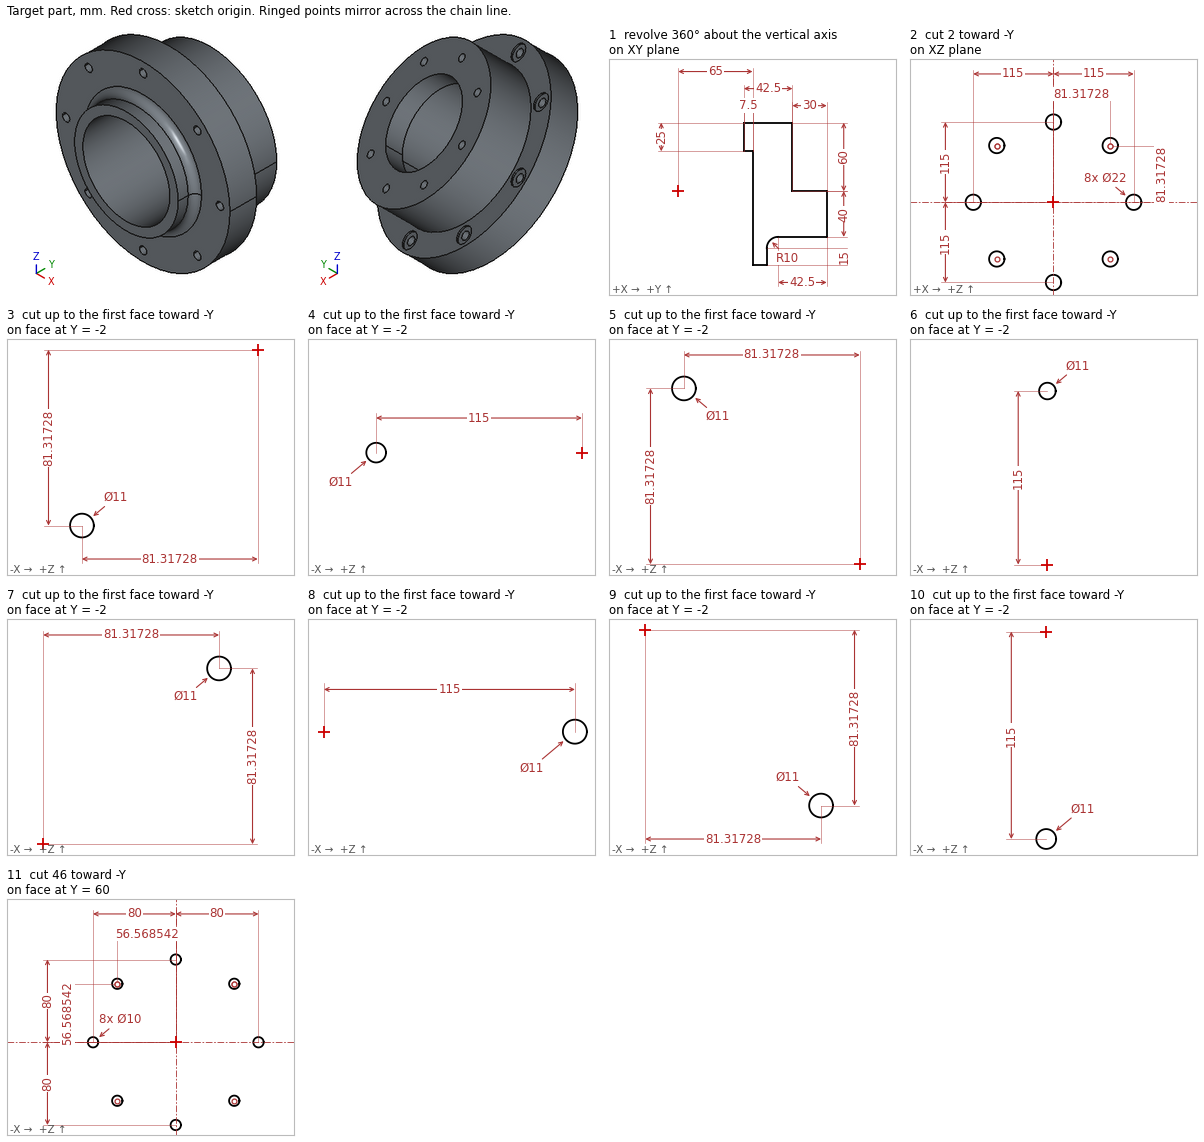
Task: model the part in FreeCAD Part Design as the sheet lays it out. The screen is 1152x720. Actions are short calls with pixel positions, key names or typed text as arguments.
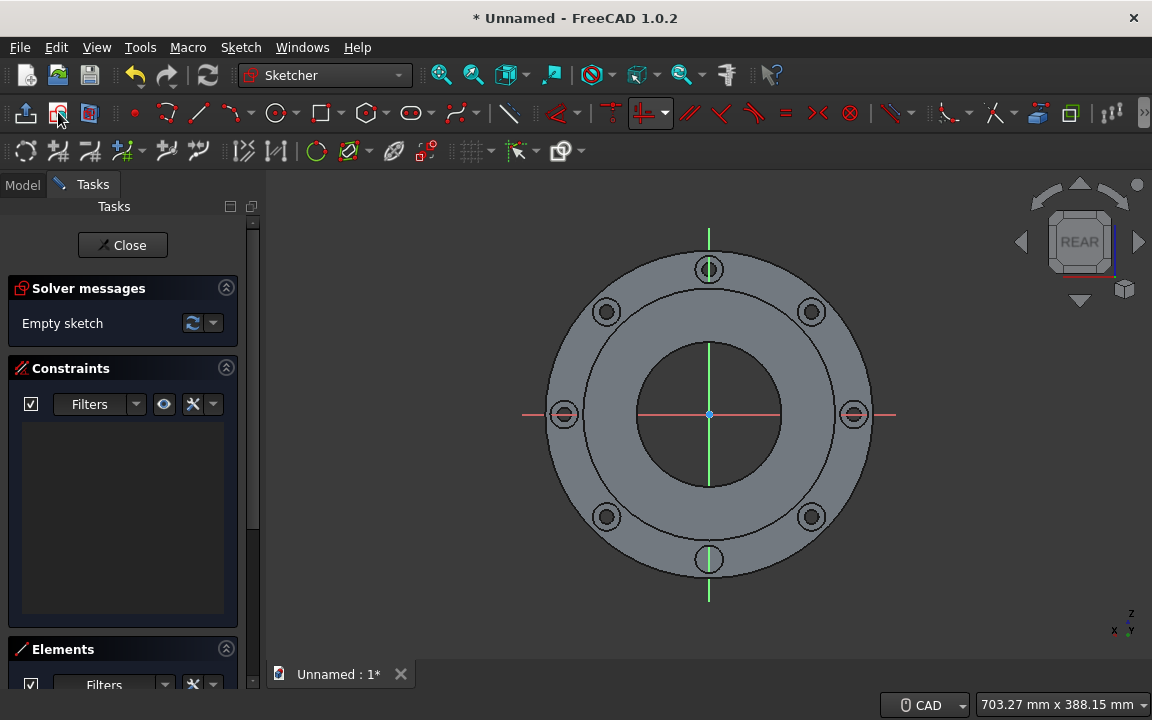
click(90, 114)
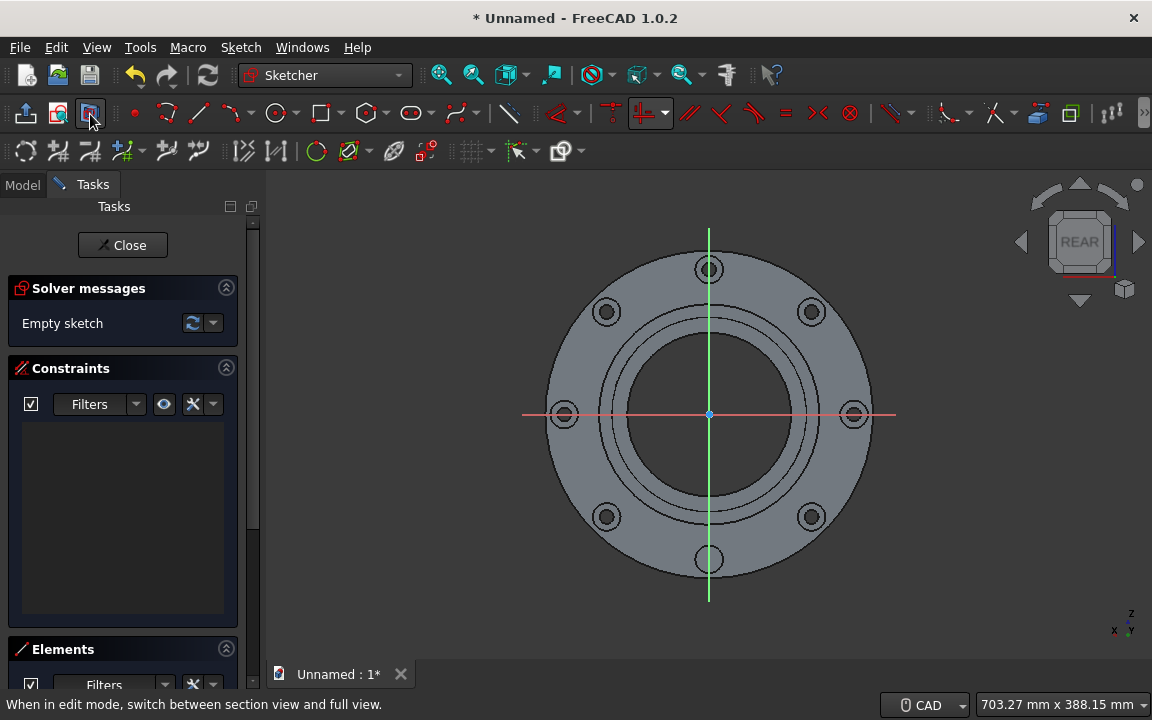
scroll(713, 567, up, 15)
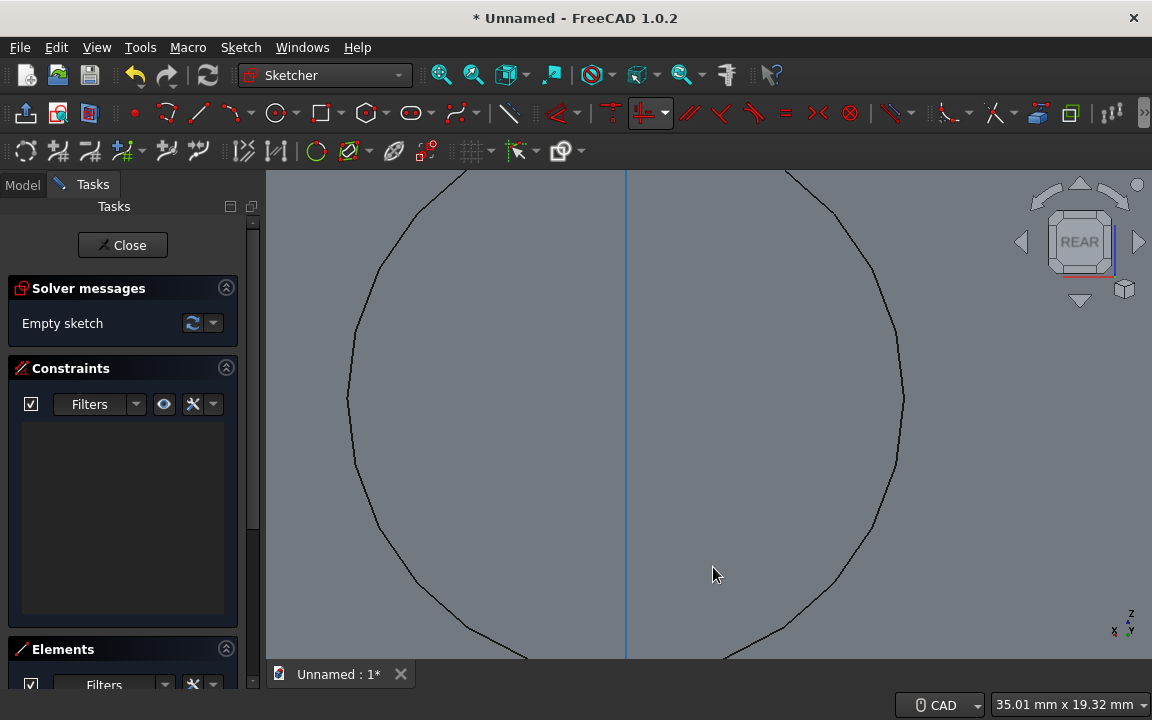
click(276, 114)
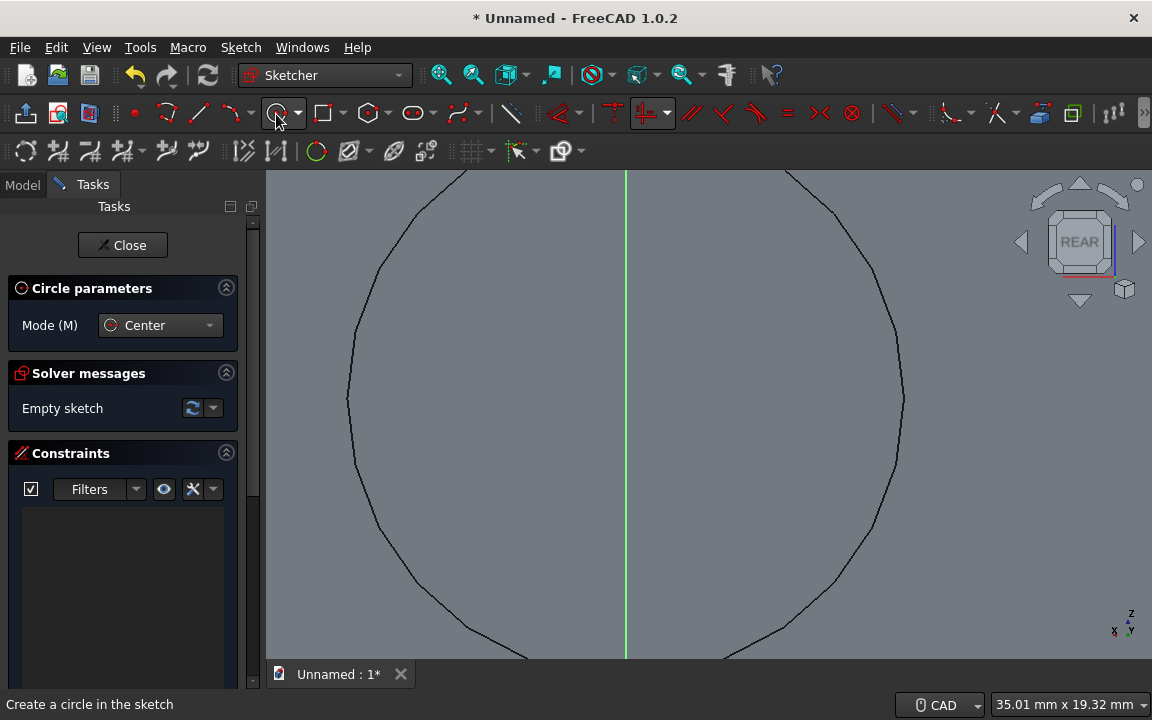
click(626, 398)
move(724, 300)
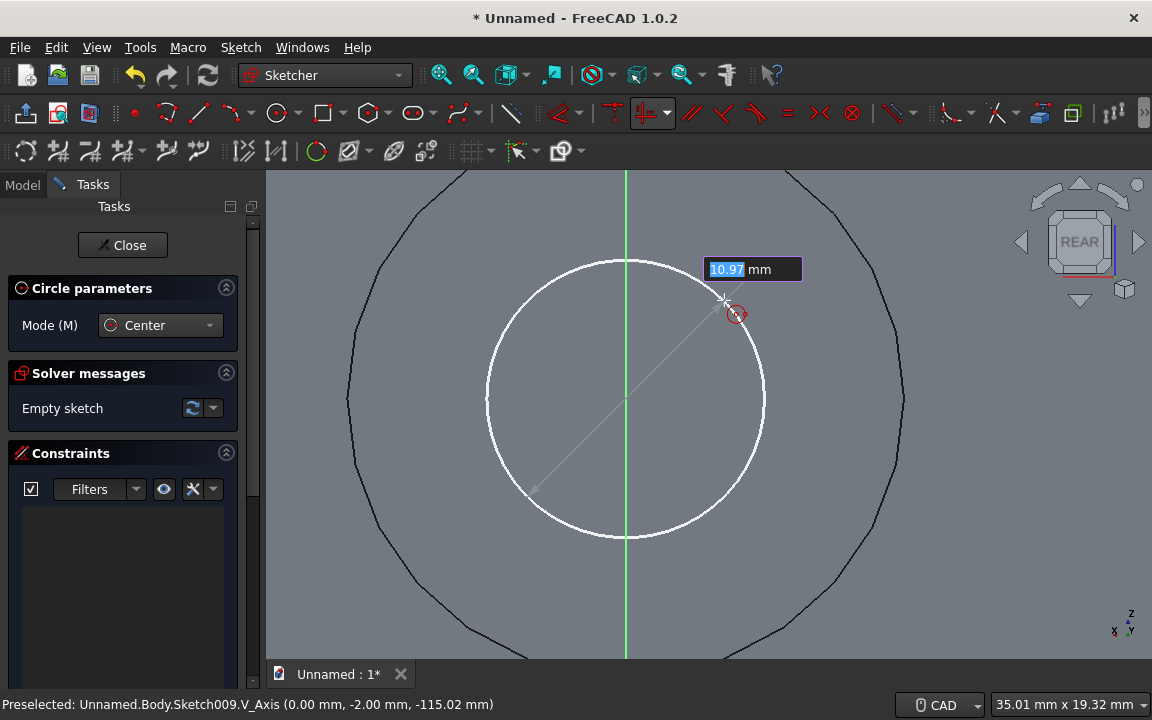
text(11)
key(Return)
key(Escape)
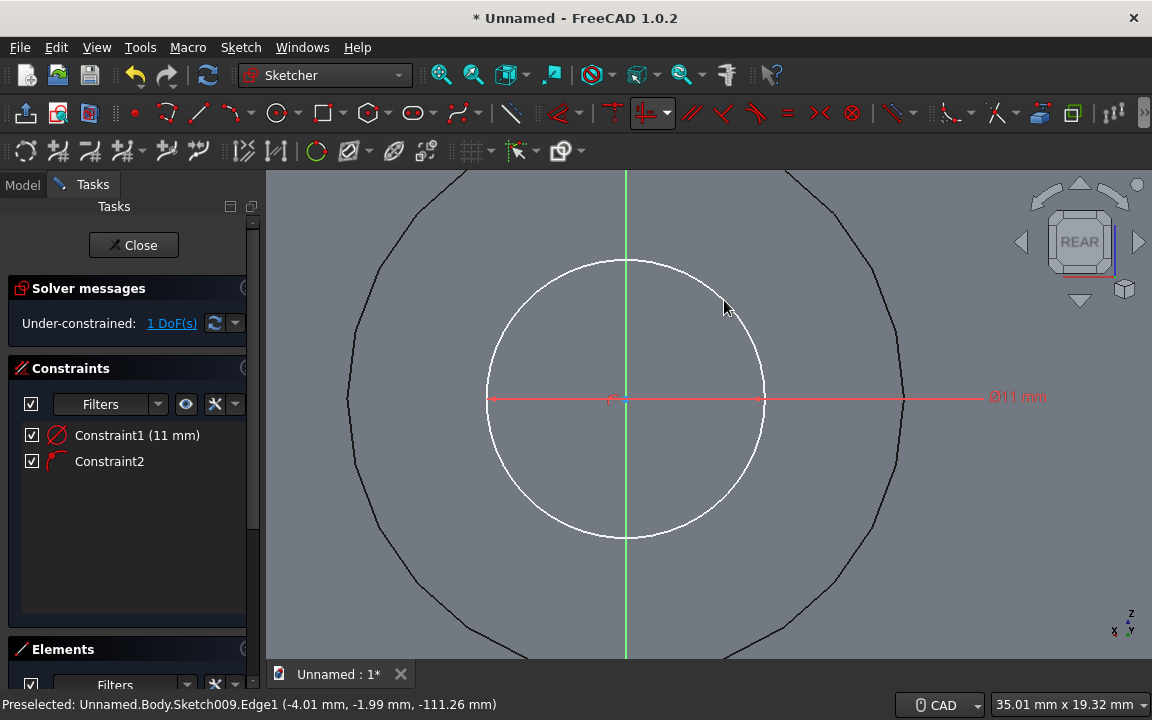
click(558, 114)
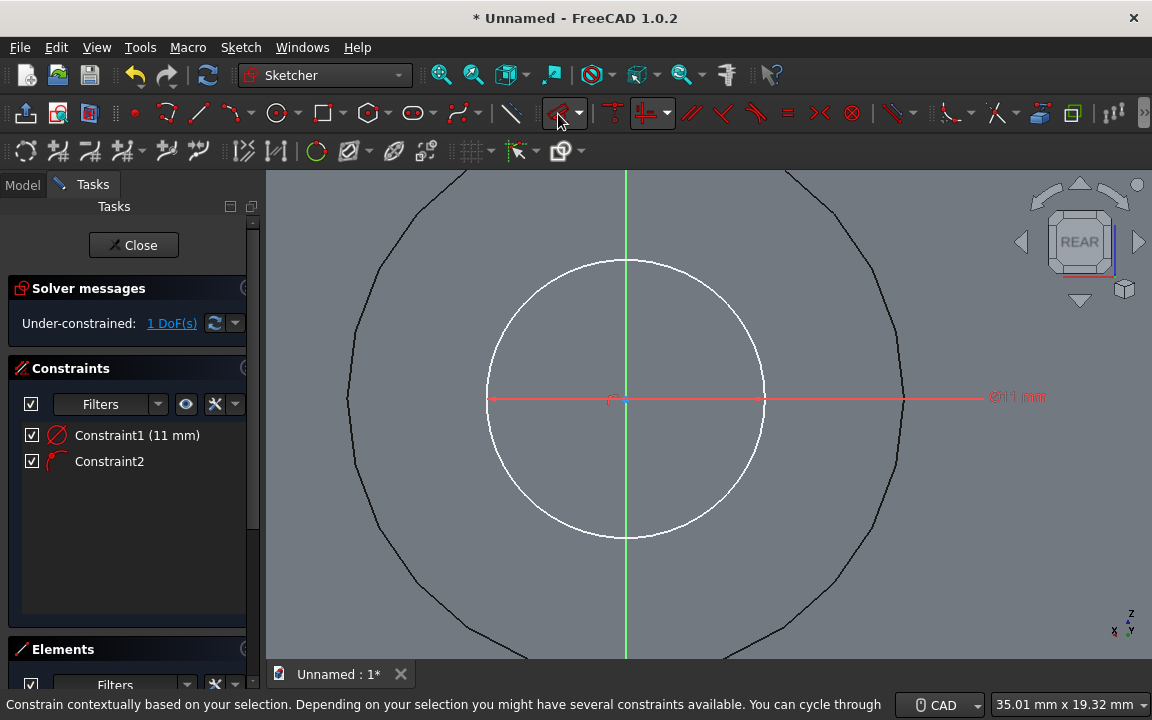
click(626, 399)
click(660, 299)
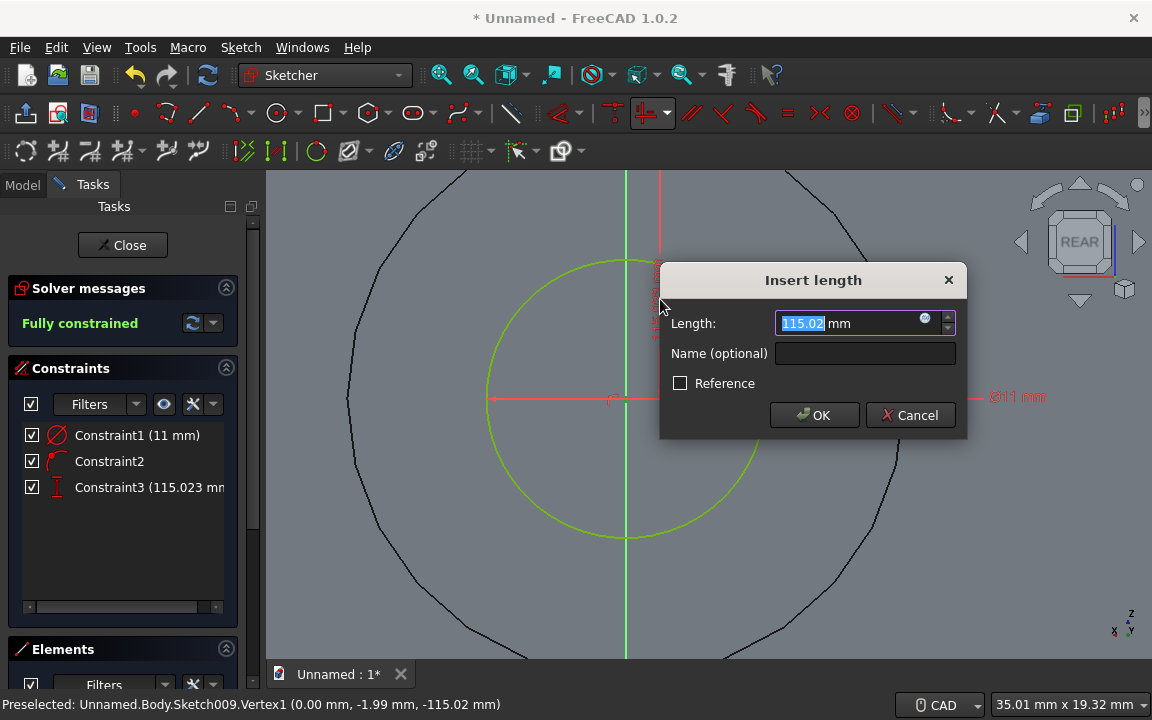
text(115)
key(Return)
key(Escape)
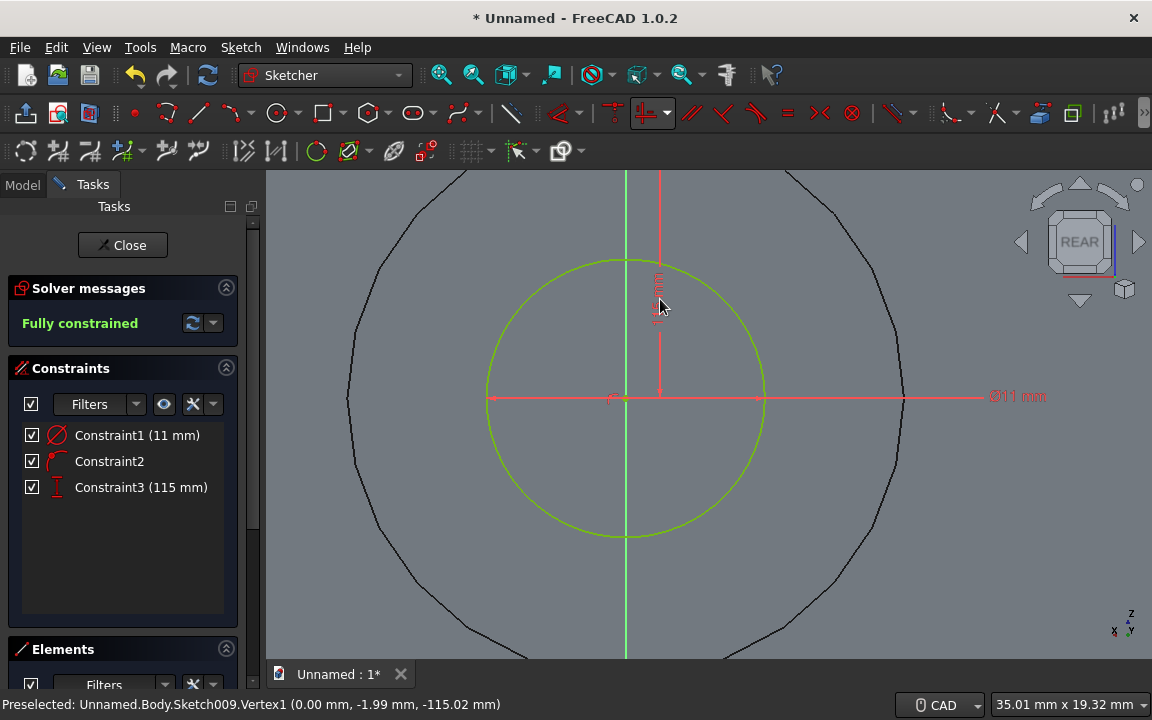
click(123, 245)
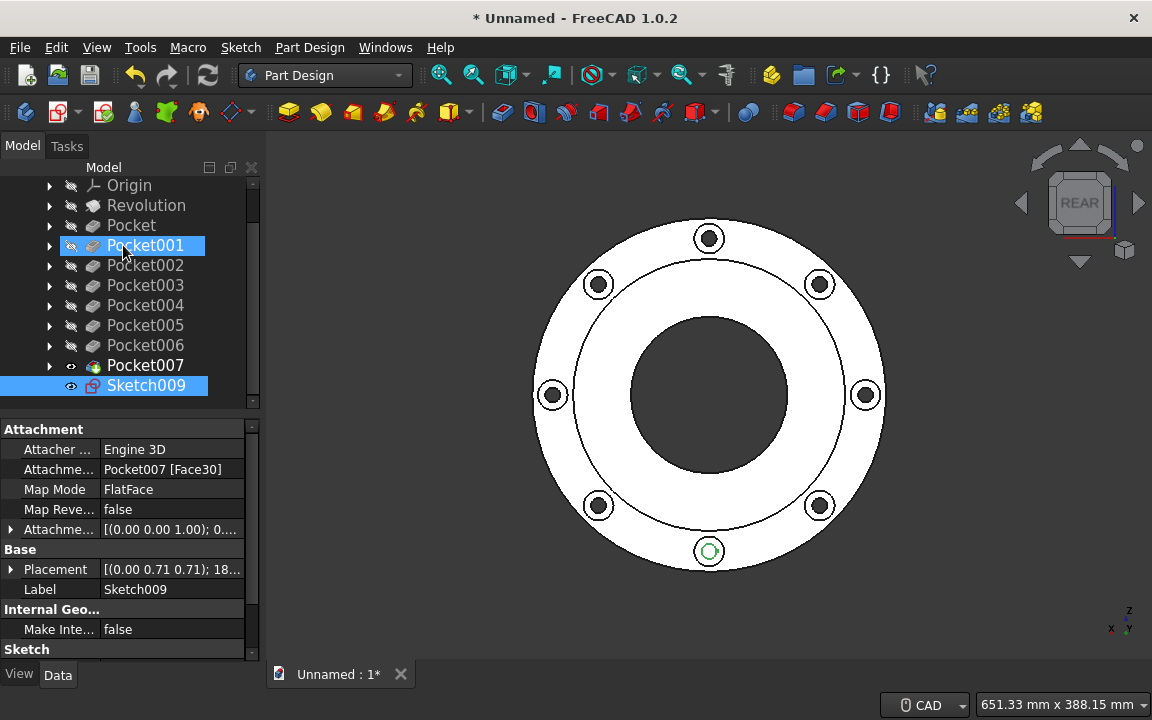
click(504, 112)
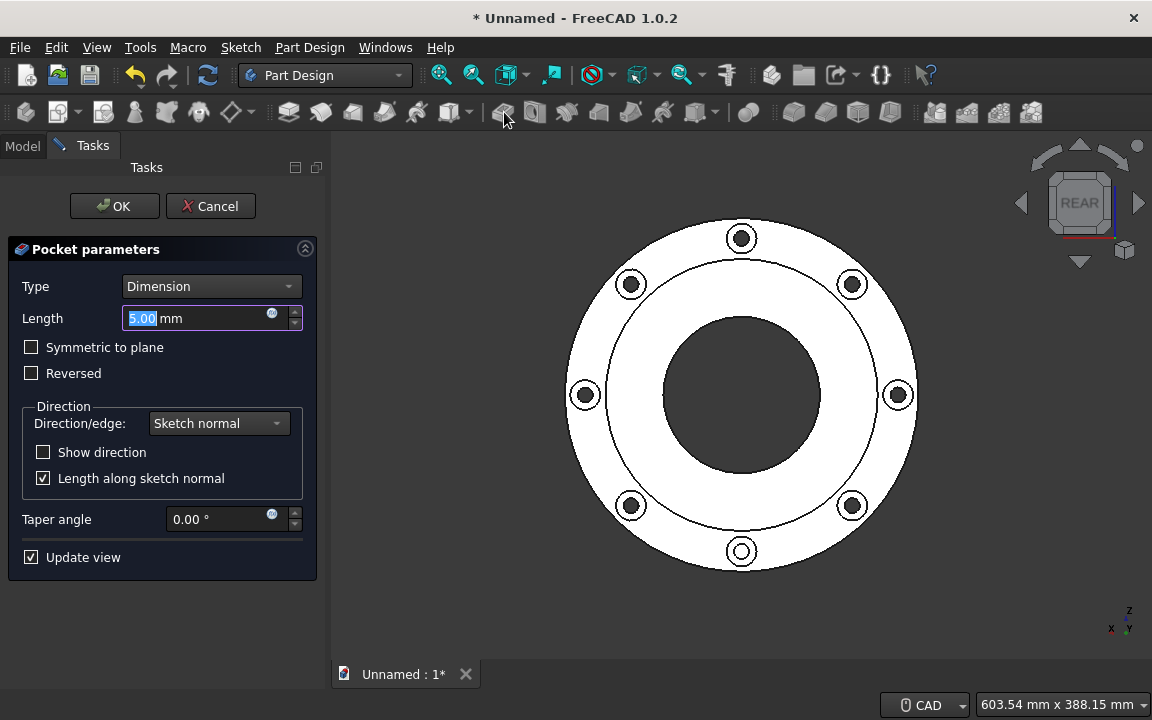
click(212, 286)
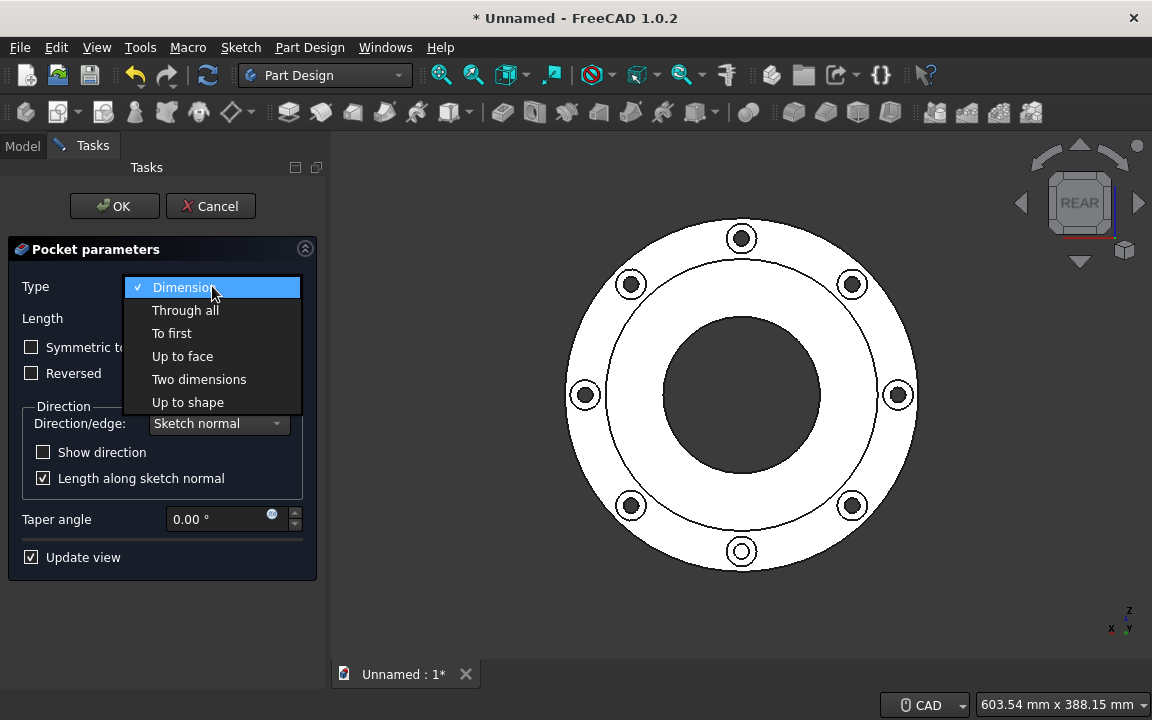
click(212, 334)